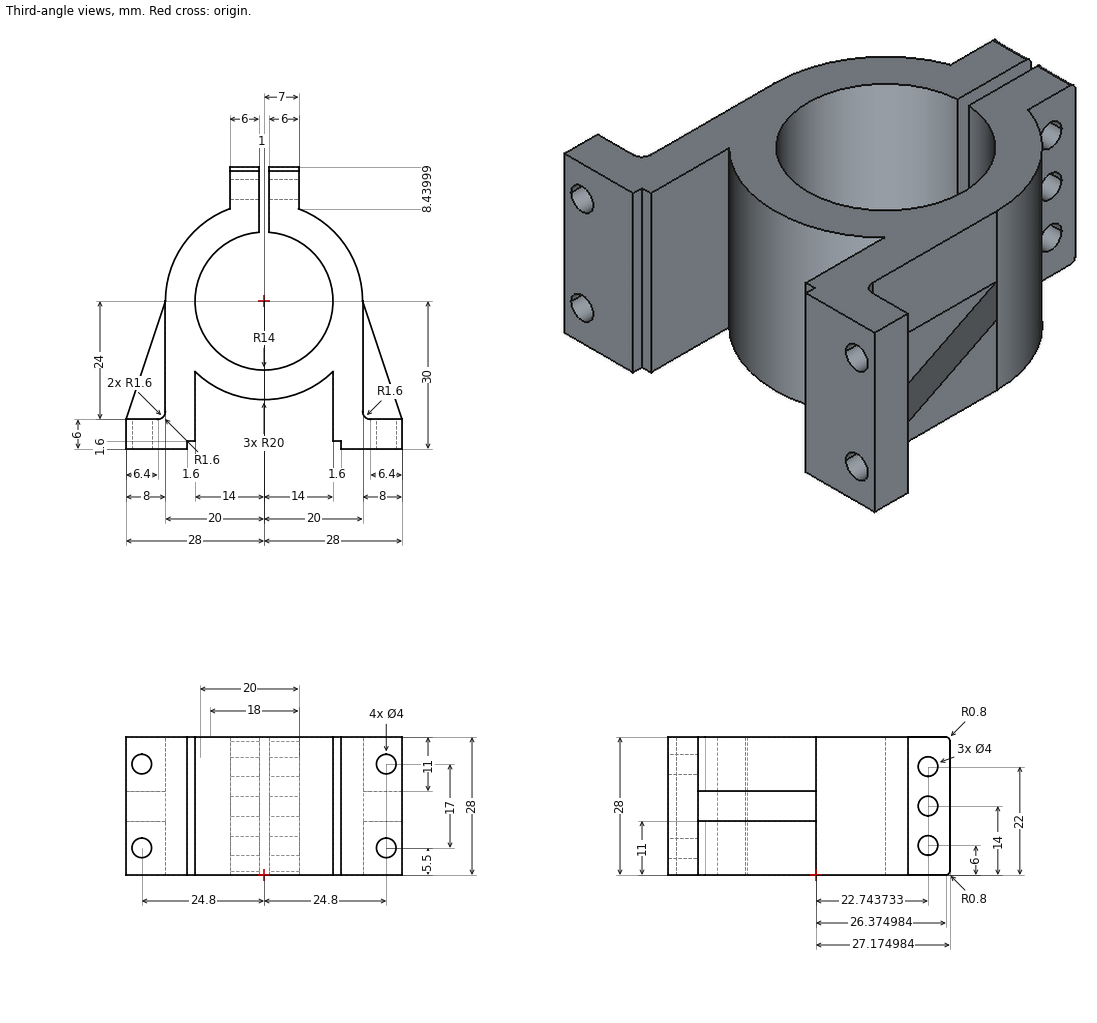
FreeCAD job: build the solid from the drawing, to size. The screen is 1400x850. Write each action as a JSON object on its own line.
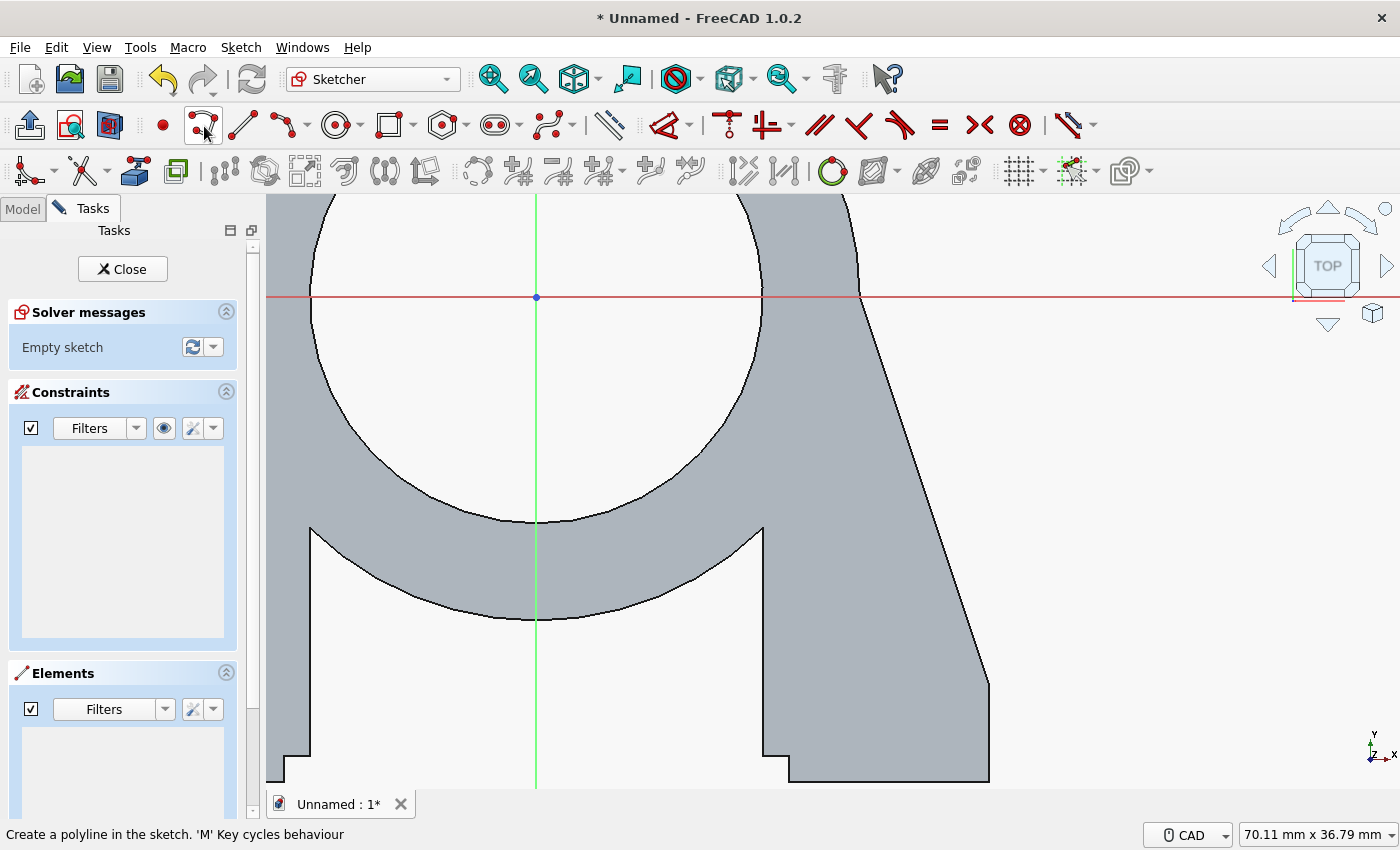
{"action": "left_click", "coordinate": [886, 685]}
{"action": "left_click", "coordinate": [989, 685]}
{"action": "left_click", "coordinate": [860, 297]}
{"action": "left_click", "coordinate": [860, 659]}
{"action": "right_click", "coordinate": [860, 659]}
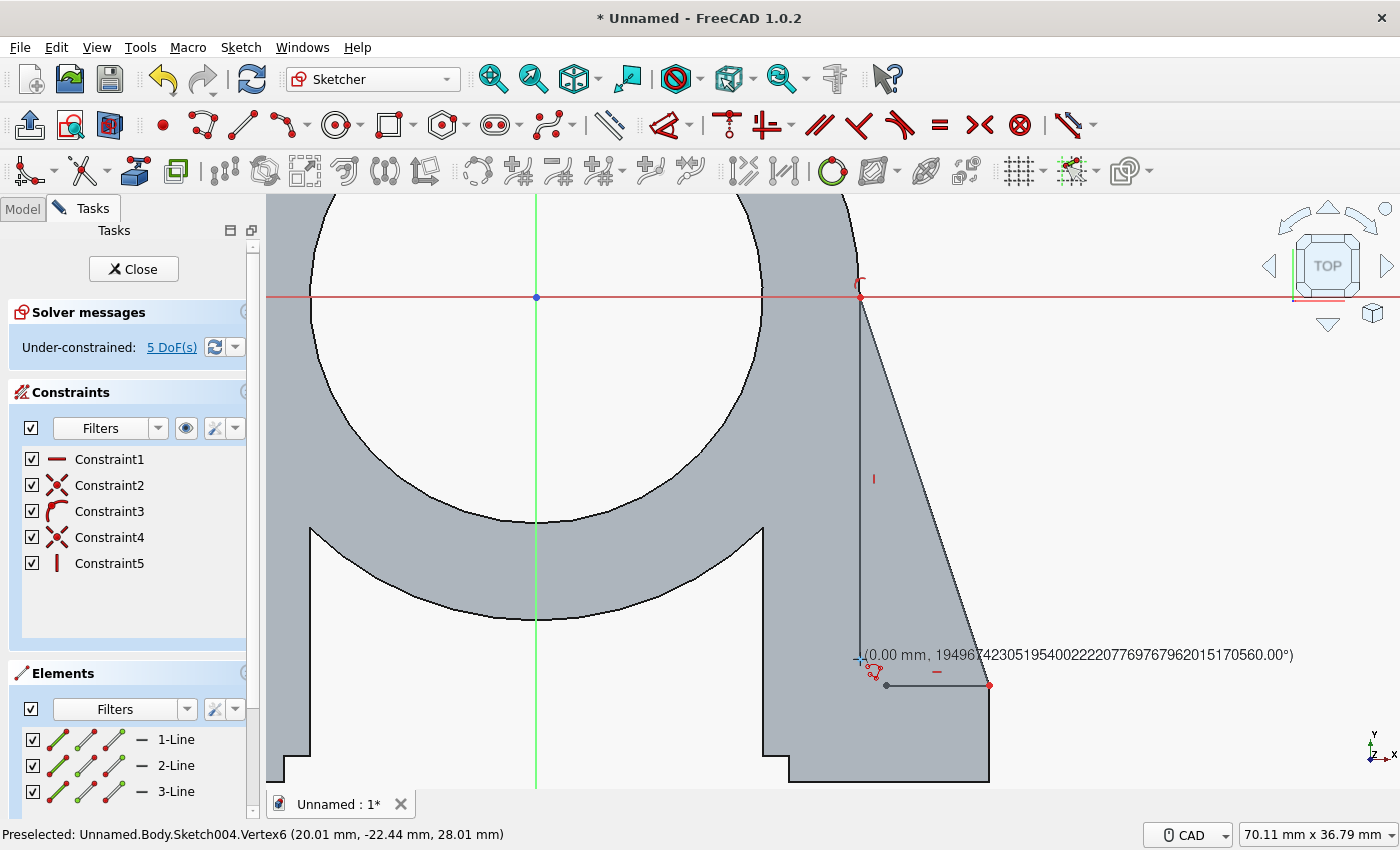
{"action": "left_click", "coordinate": [284, 126]}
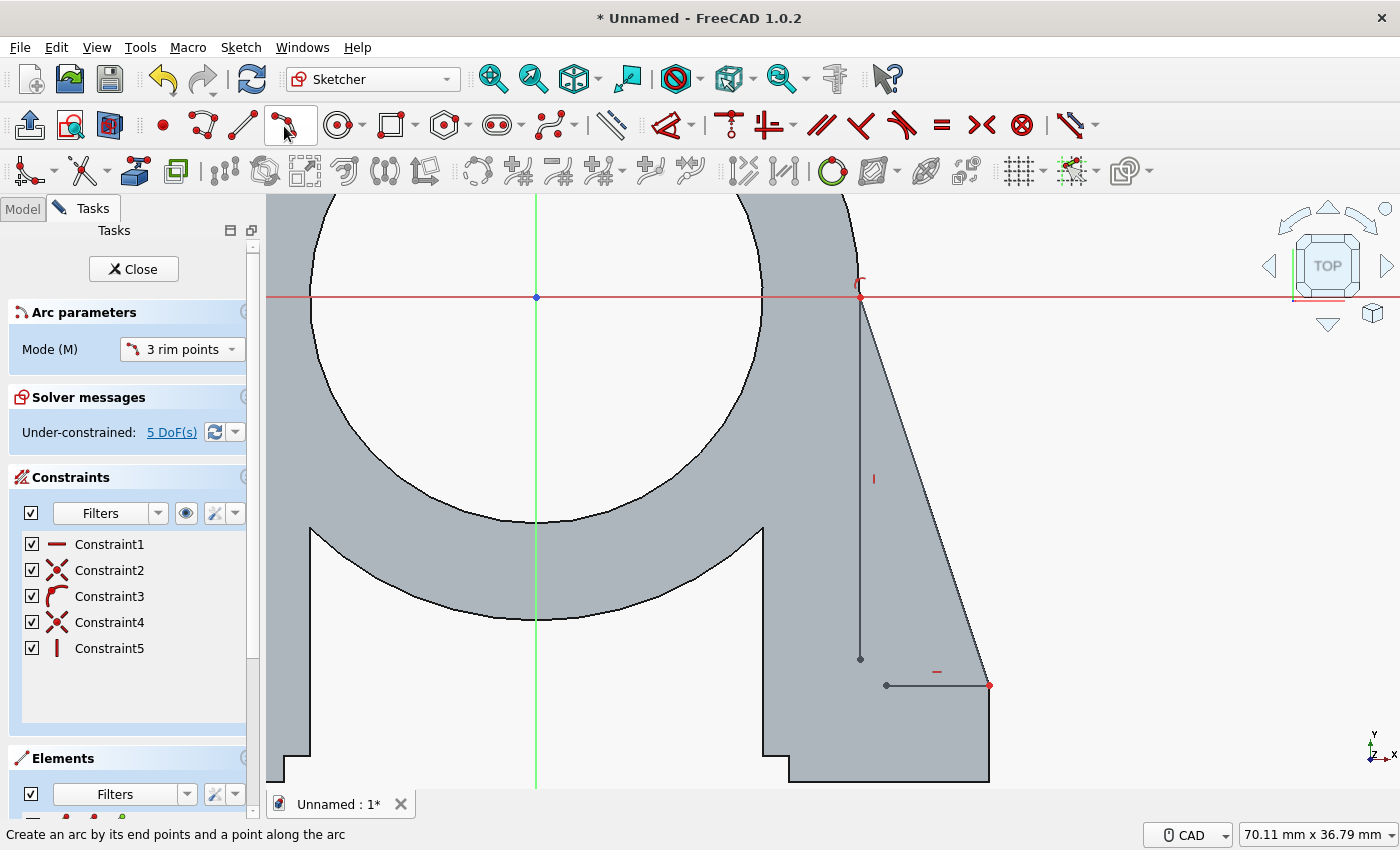
{"action": "left_click", "coordinate": [860, 660]}
{"action": "left_click", "coordinate": [886, 686]}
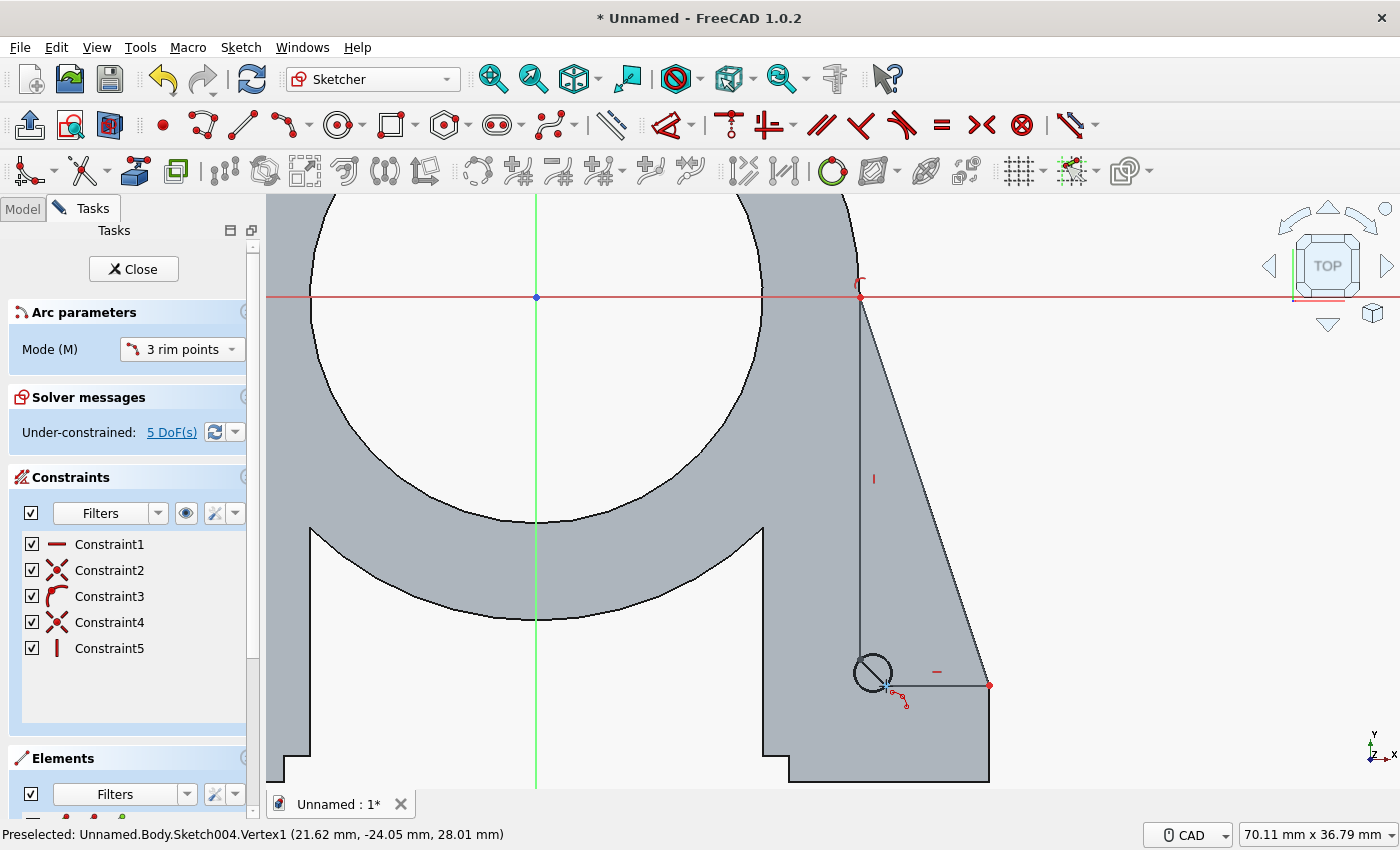
{"action": "scroll", "coordinate": [867, 678], "scroll_direction": "up", "scroll_amount": 4}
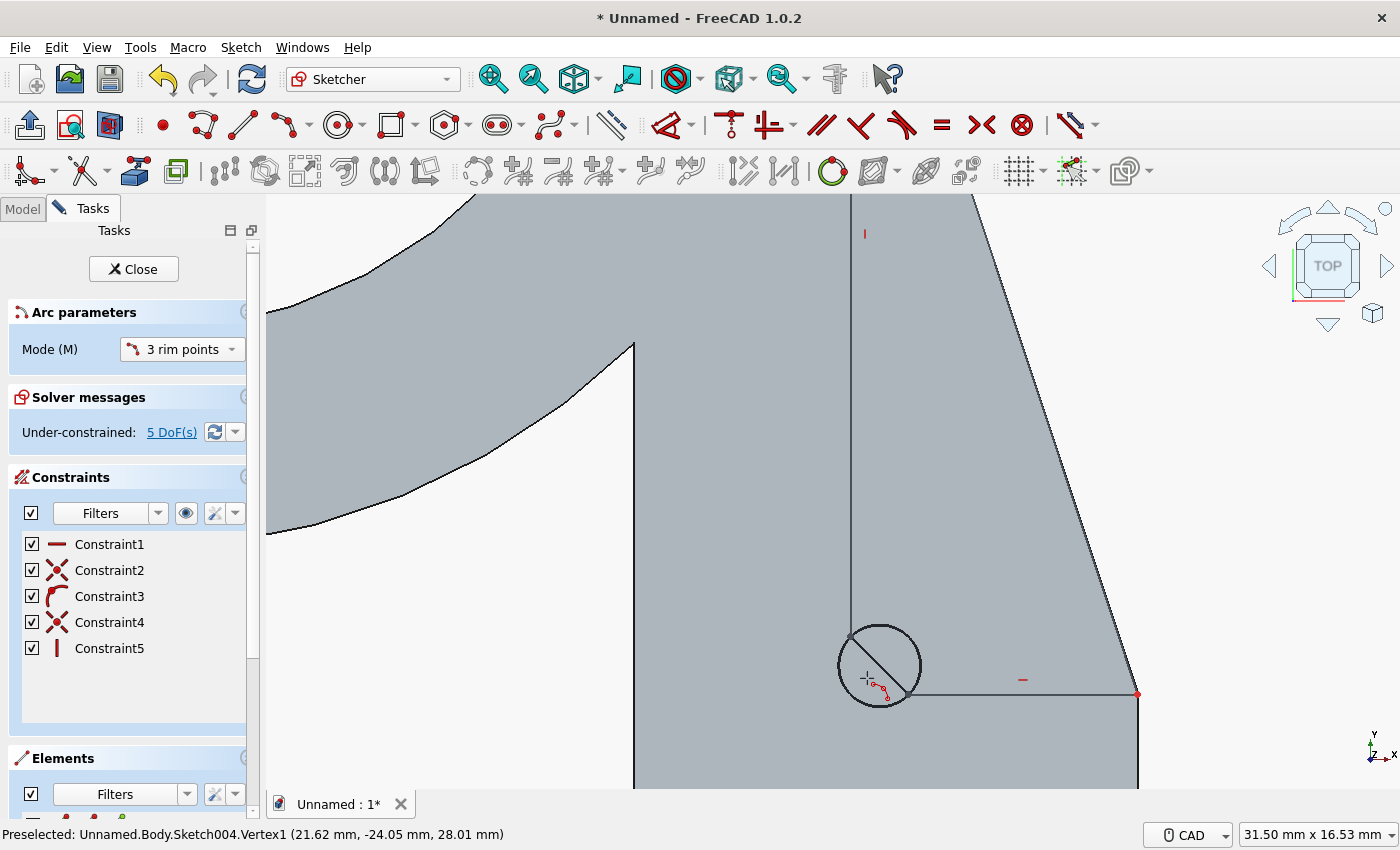
{"action": "left_click", "coordinate": [867, 676]}
{"action": "key", "text": "Escape"}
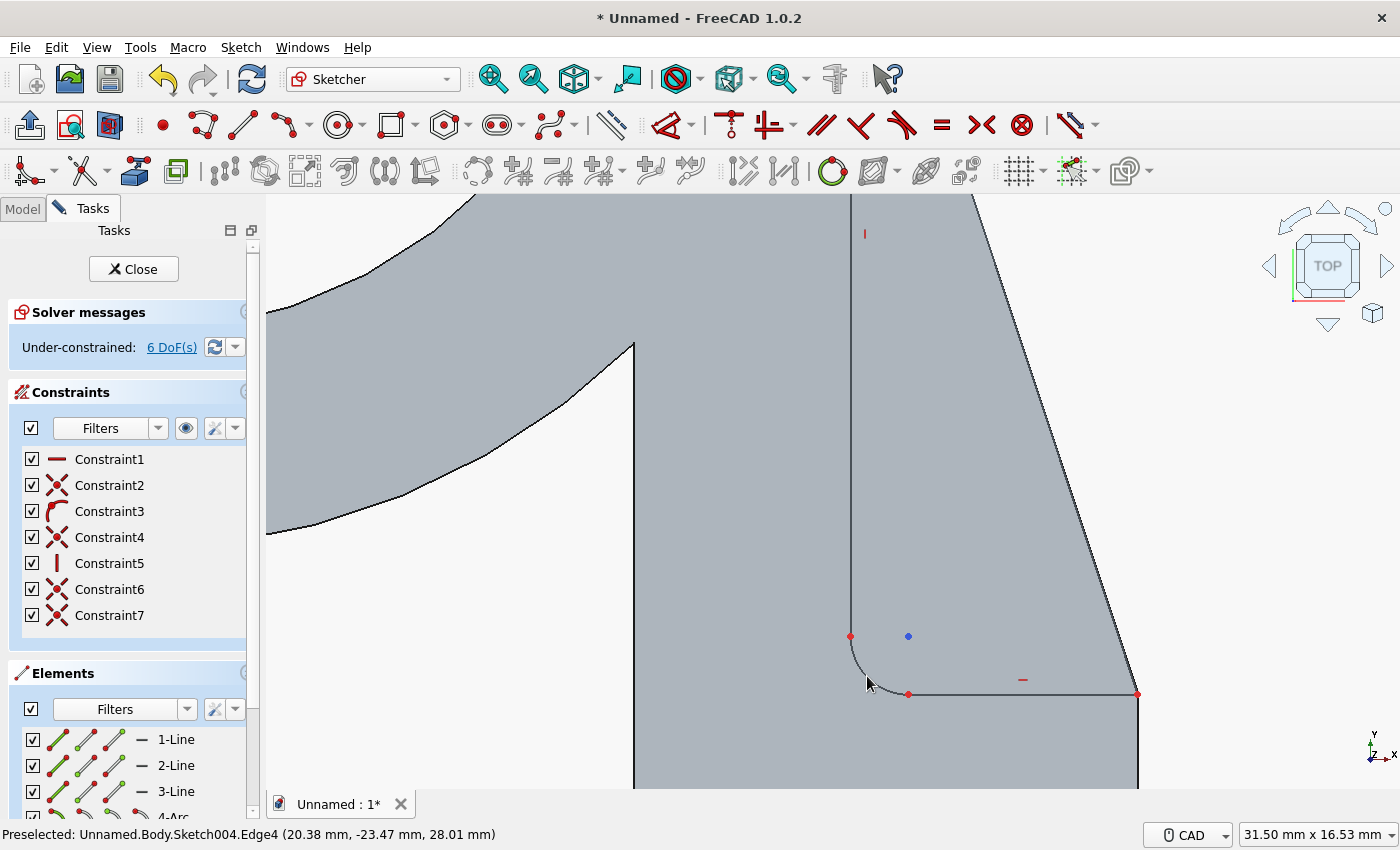
{"action": "left_click", "coordinate": [977, 695]}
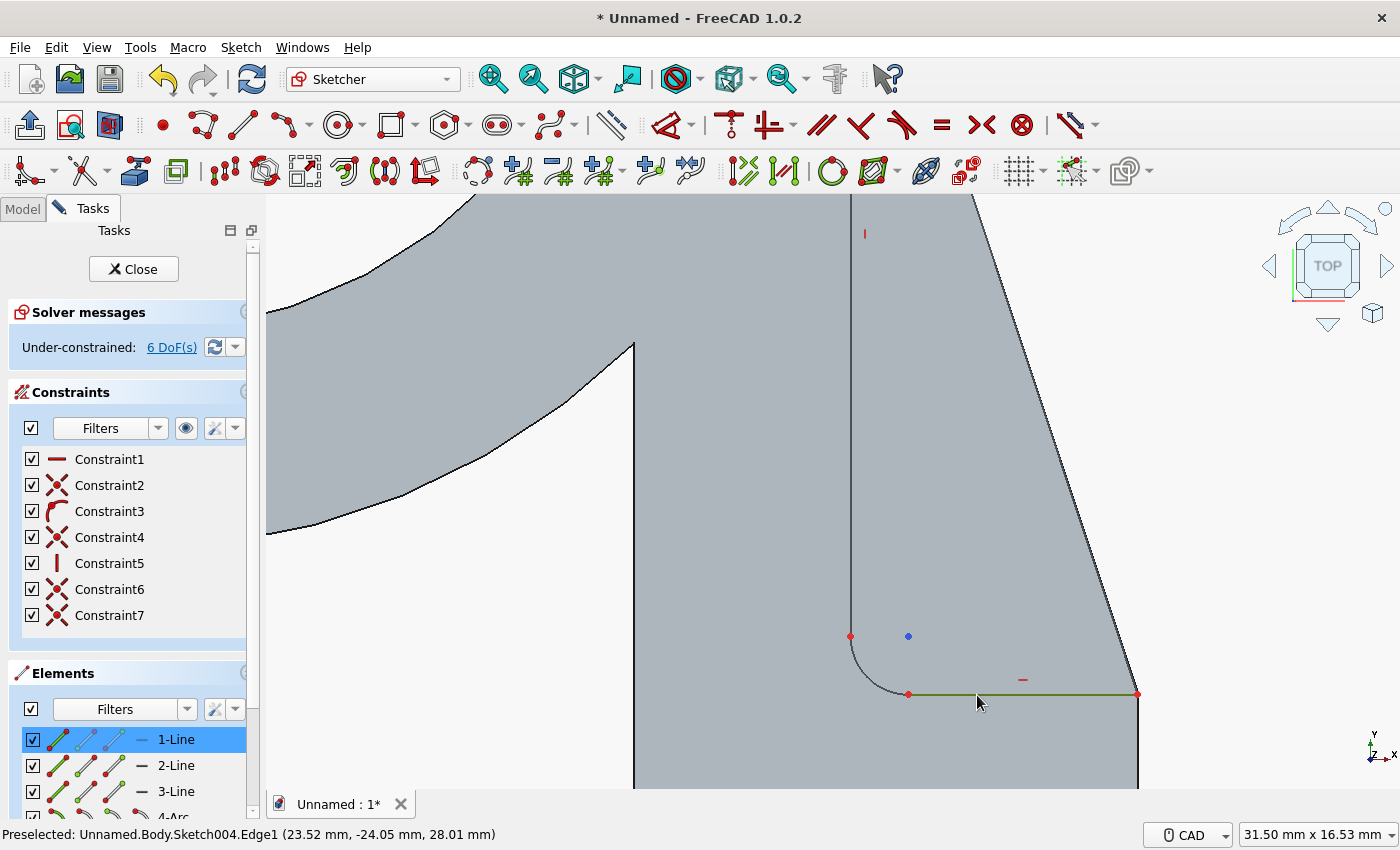
{"action": "left_click", "coordinate": [857, 663]}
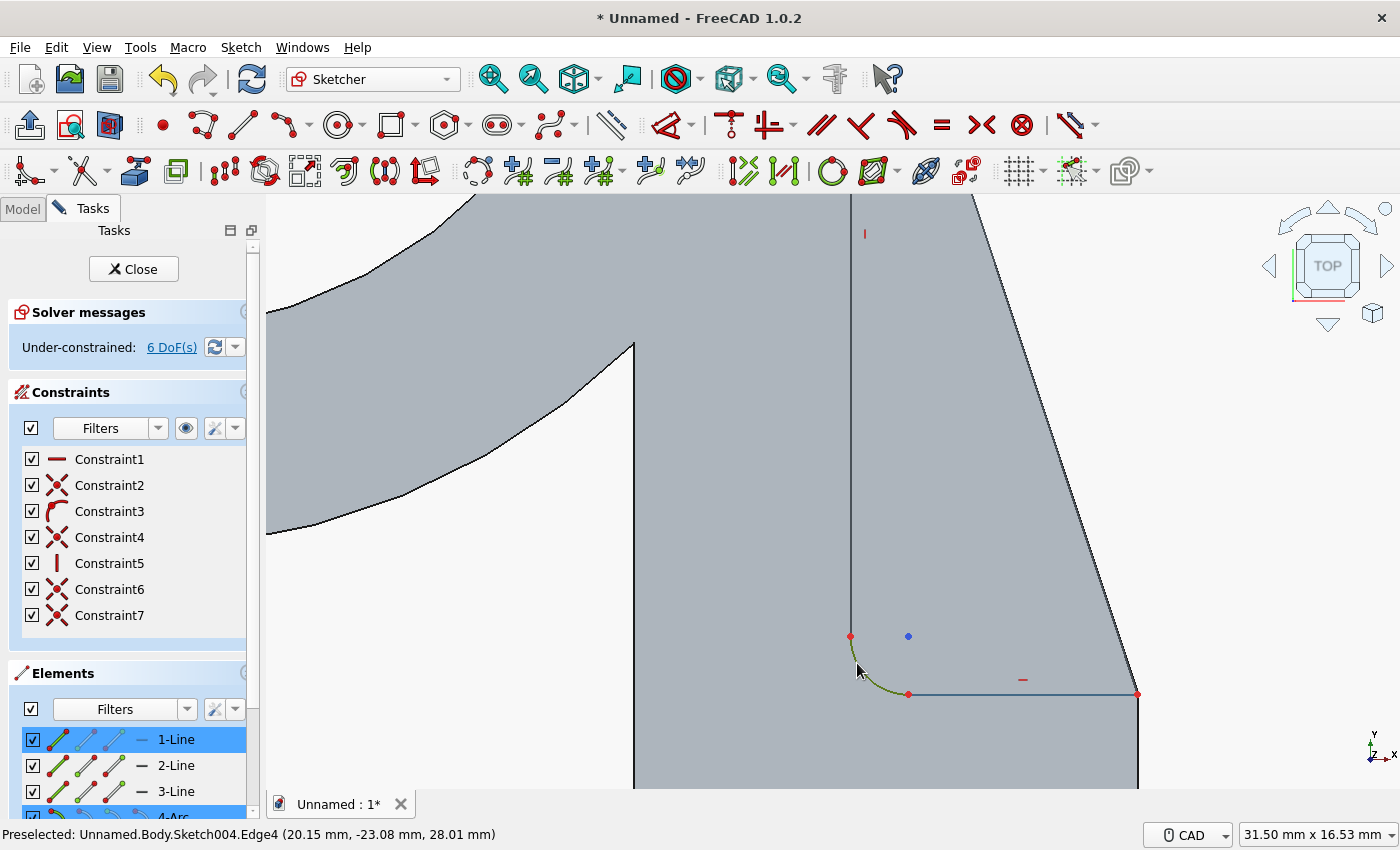
{"action": "left_click", "coordinate": [902, 126]}